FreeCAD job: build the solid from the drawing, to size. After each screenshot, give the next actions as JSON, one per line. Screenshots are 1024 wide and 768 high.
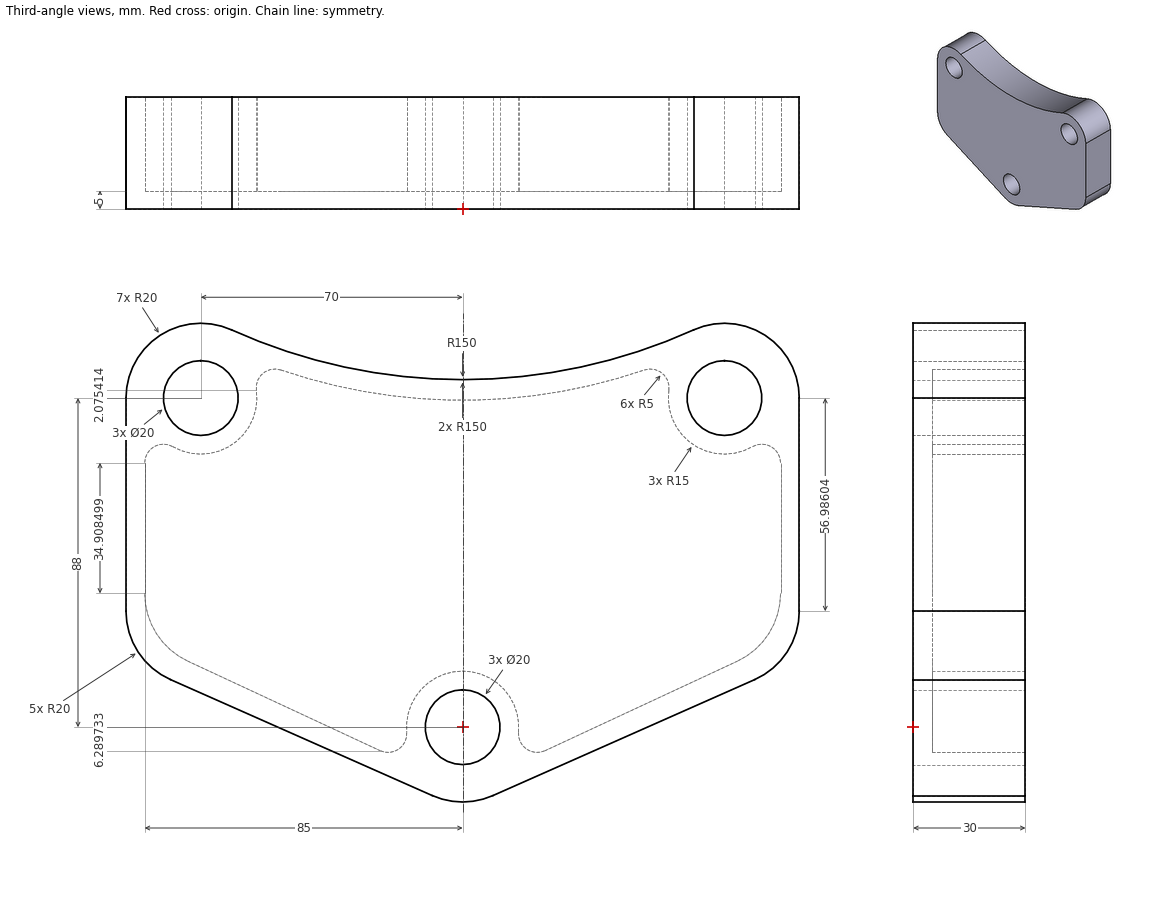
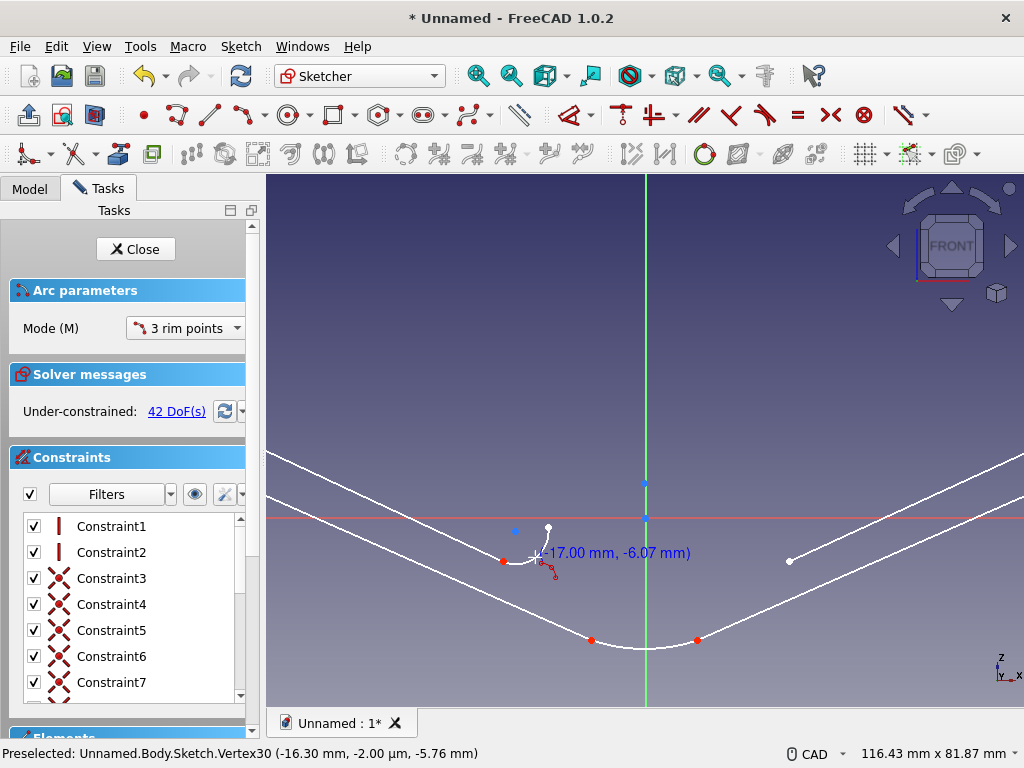
{"action": "scroll", "coordinate": [548, 527], "scroll_direction": "up", "scroll_amount": 4}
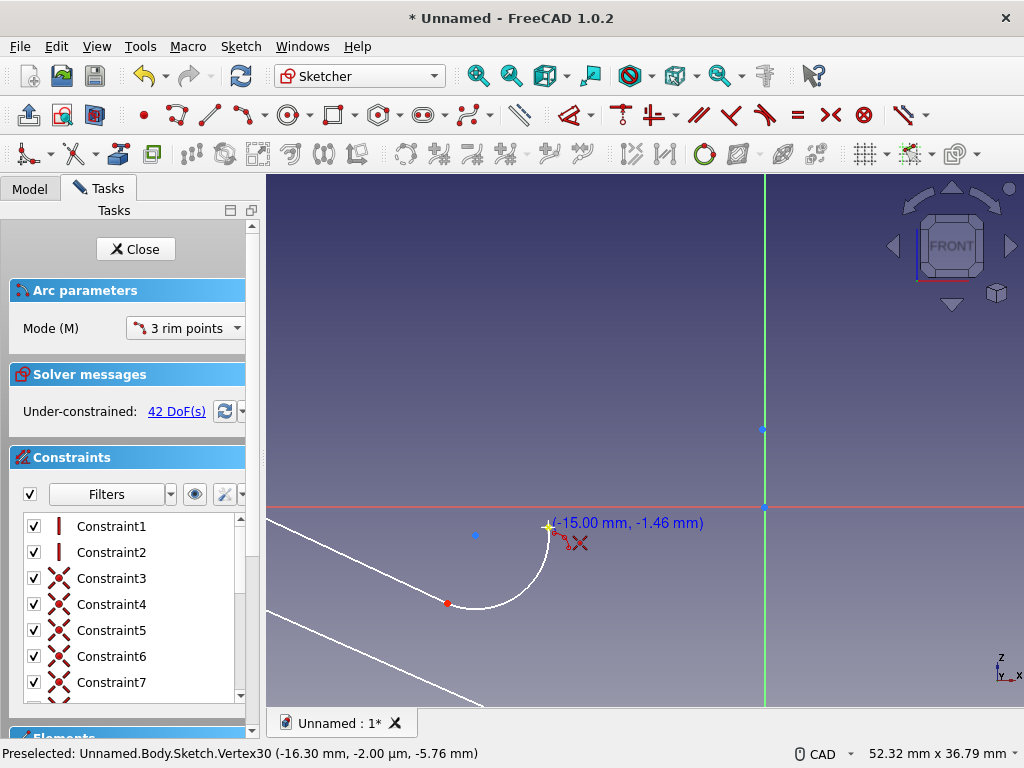
{"action": "left_click", "coordinate": [548, 527]}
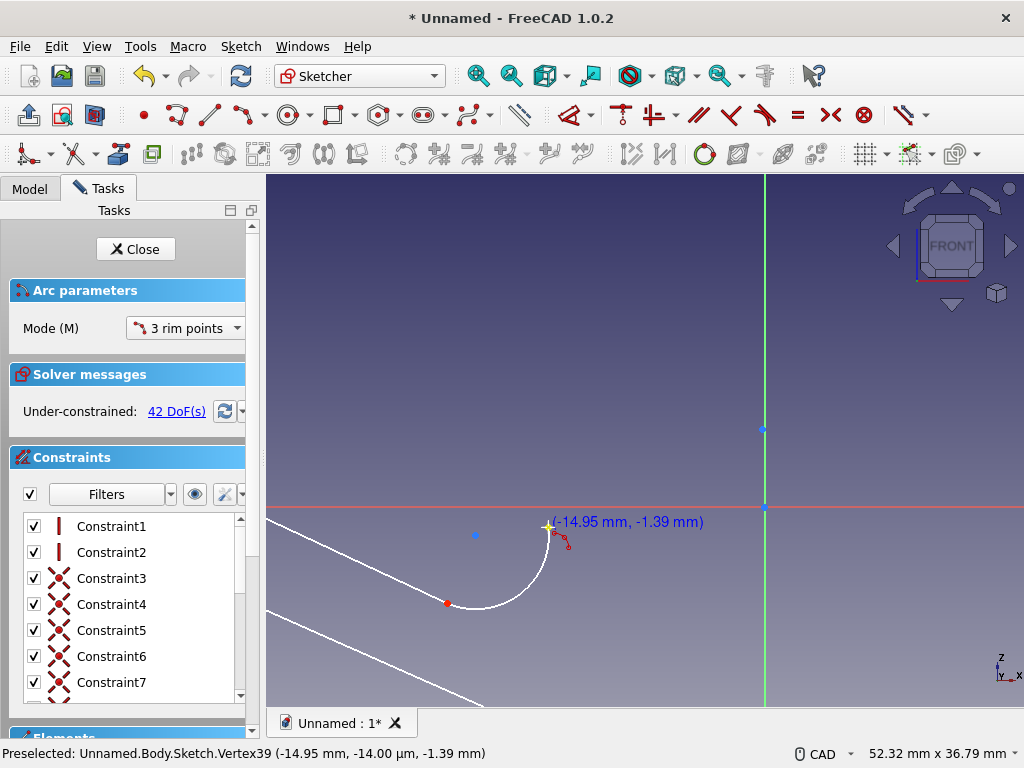
{"action": "scroll", "coordinate": [539, 551], "scroll_direction": "down", "scroll_amount": 9}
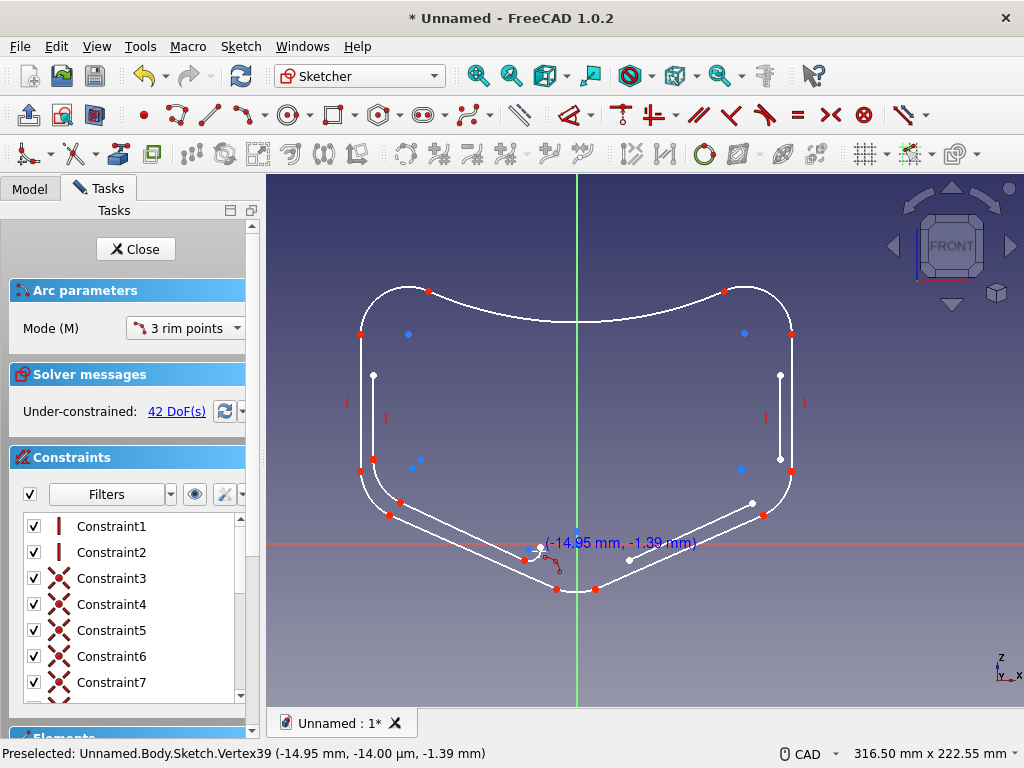
{"action": "scroll", "coordinate": [612, 548], "scroll_direction": "up", "scroll_amount": 9}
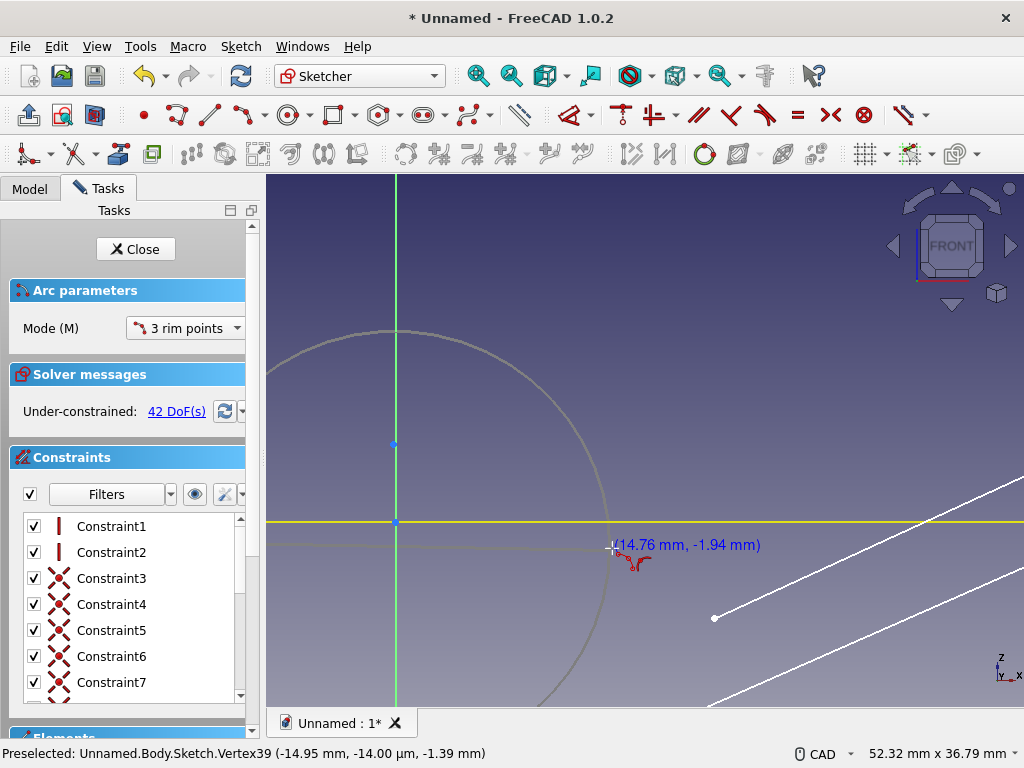
{"action": "left_click", "coordinate": [612, 541]}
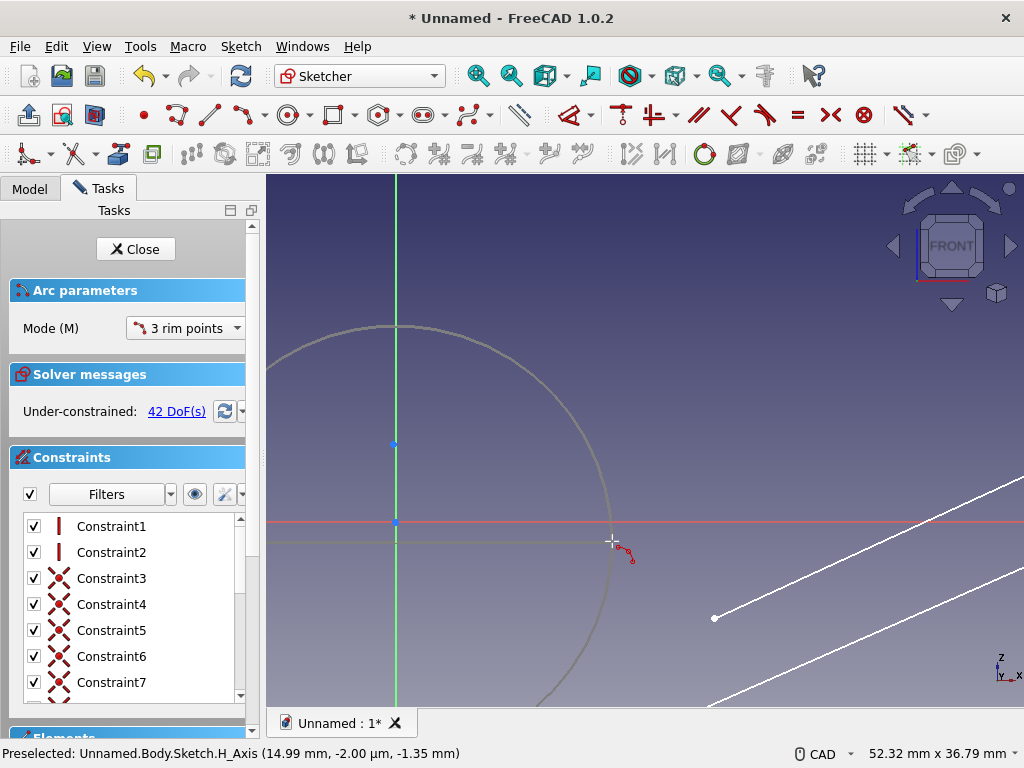
{"action": "scroll", "coordinate": [612, 548], "scroll_direction": "down", "scroll_amount": 9}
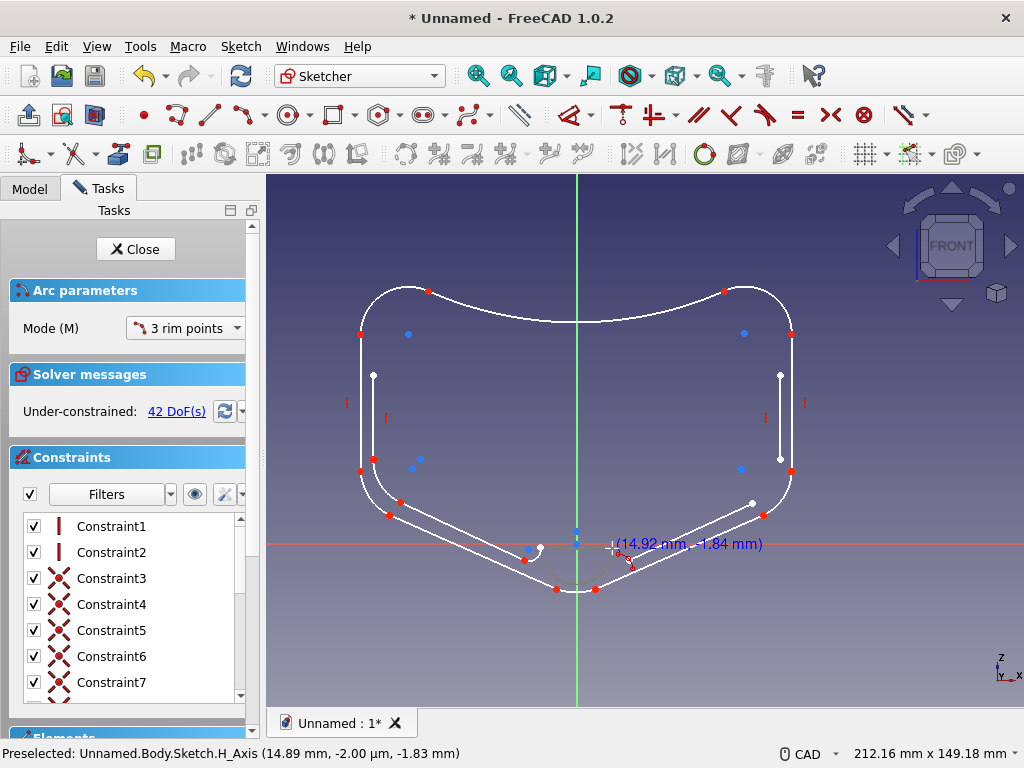
{"action": "left_click", "coordinate": [599, 516]}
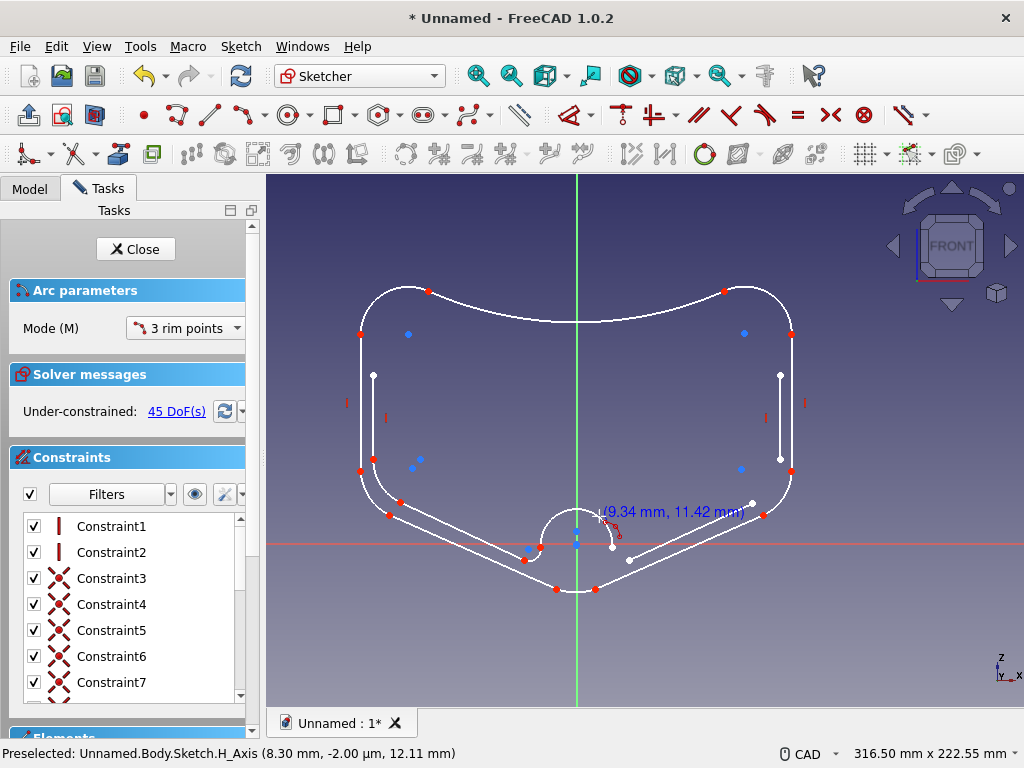
{"action": "scroll", "coordinate": [612, 548], "scroll_direction": "up", "scroll_amount": 9}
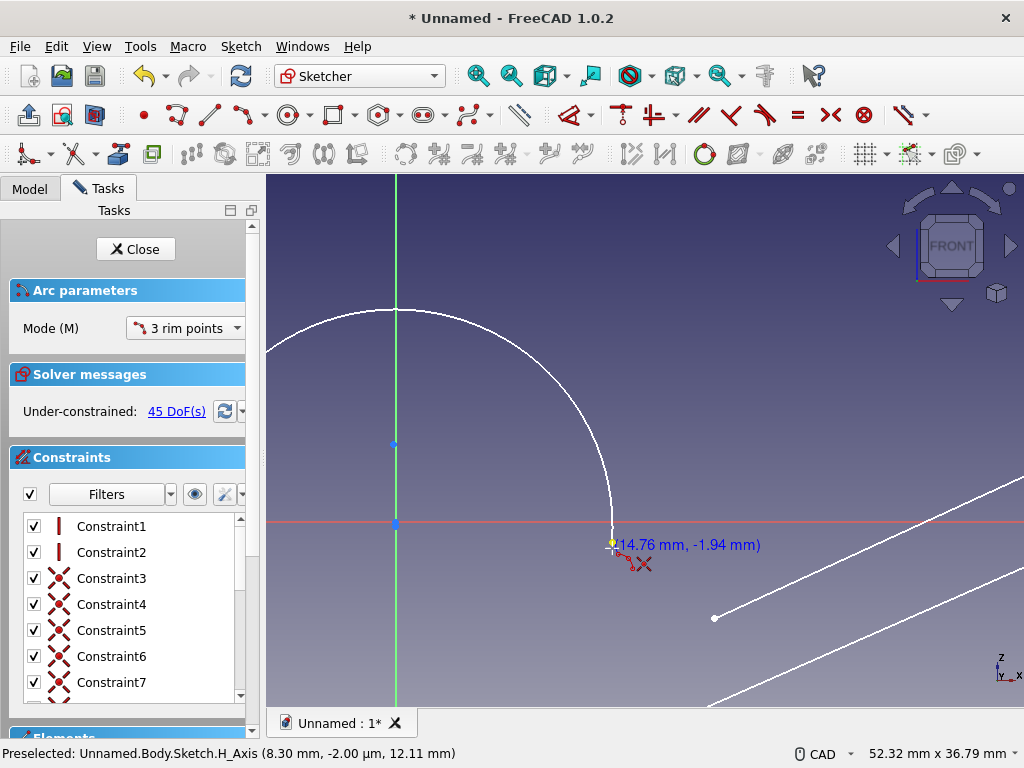
{"action": "left_click", "coordinate": [612, 542]}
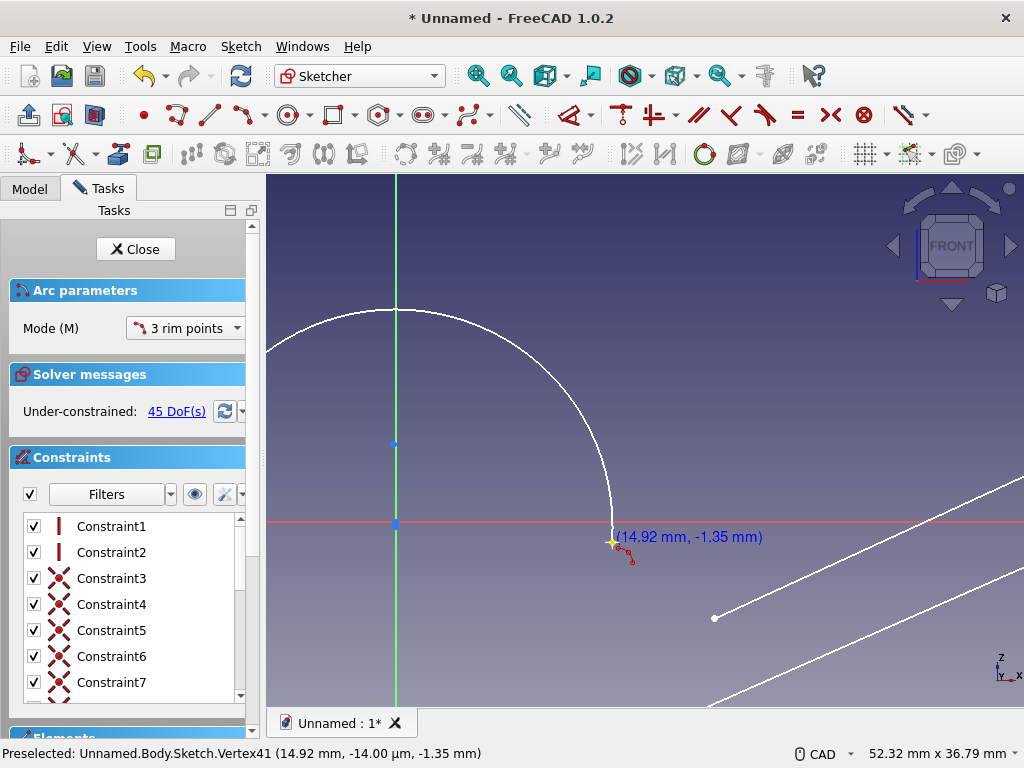
{"action": "scroll", "coordinate": [612, 548], "scroll_direction": "down", "scroll_amount": 9}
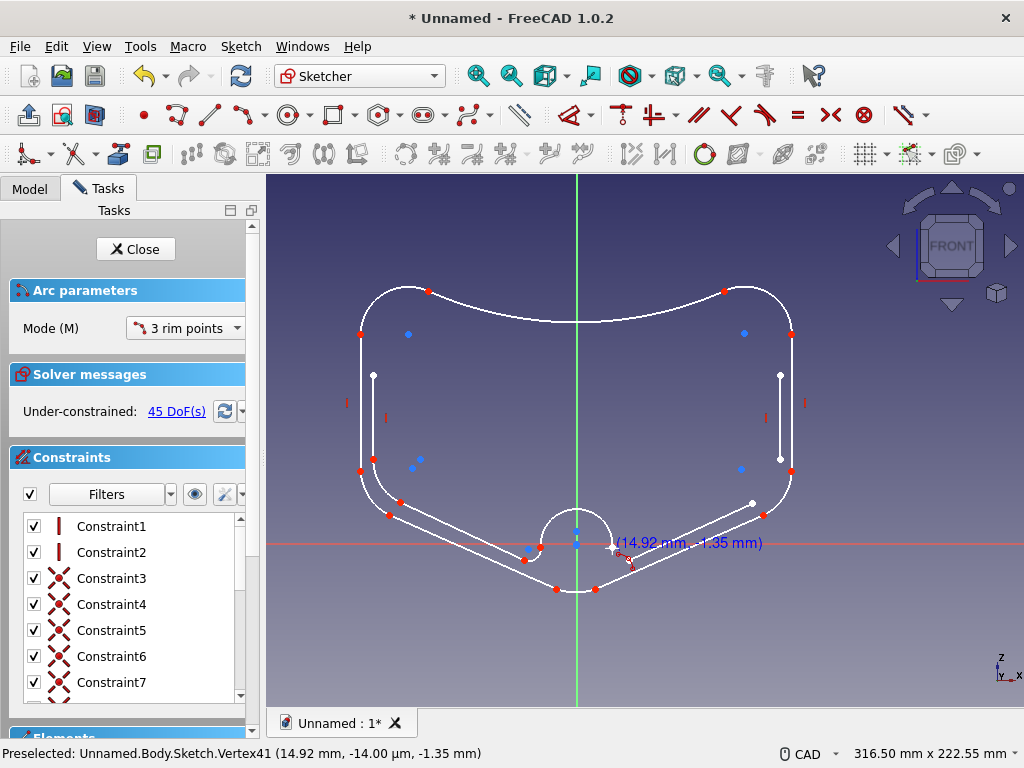
{"action": "scroll", "coordinate": [629, 559], "scroll_direction": "up", "scroll_amount": 2}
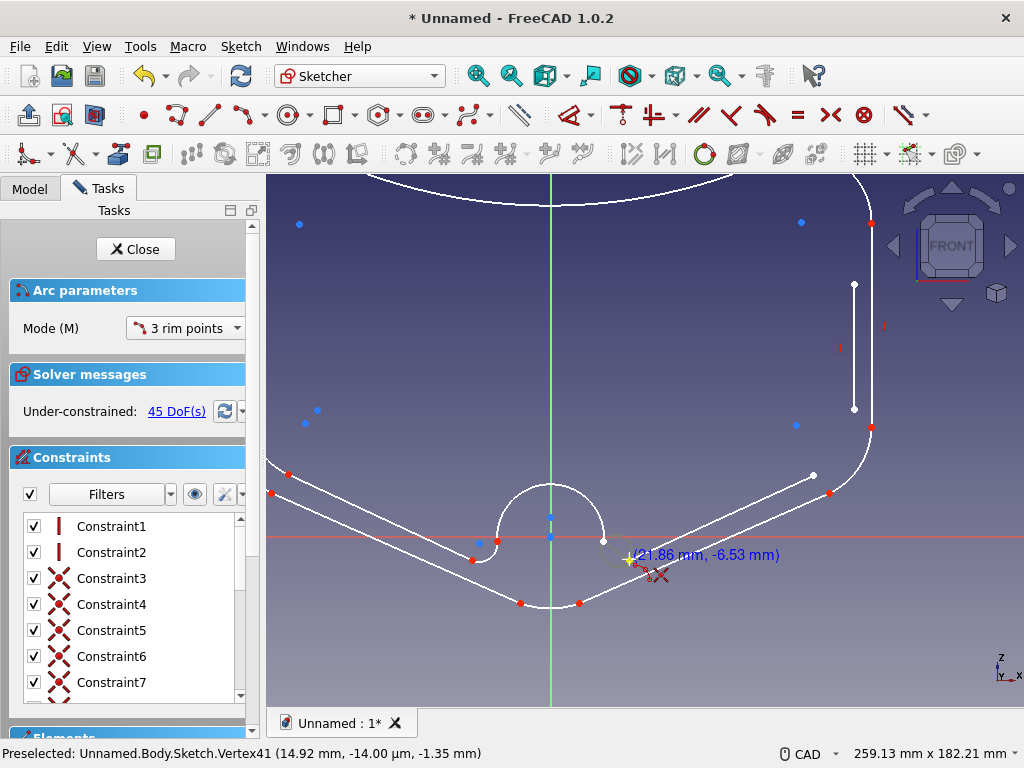
{"action": "left_click", "coordinate": [629, 561]}